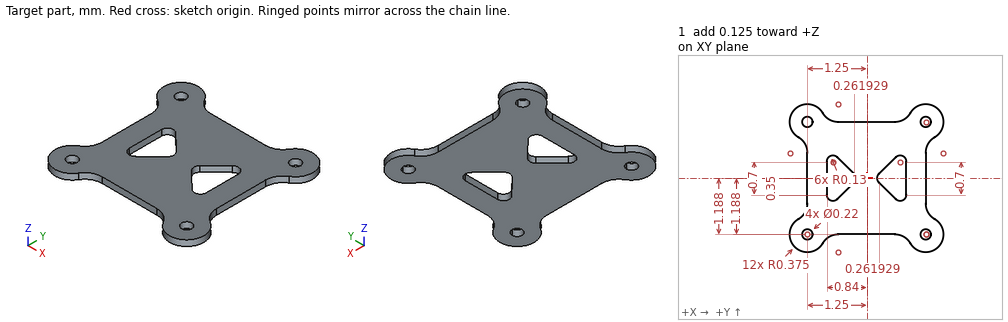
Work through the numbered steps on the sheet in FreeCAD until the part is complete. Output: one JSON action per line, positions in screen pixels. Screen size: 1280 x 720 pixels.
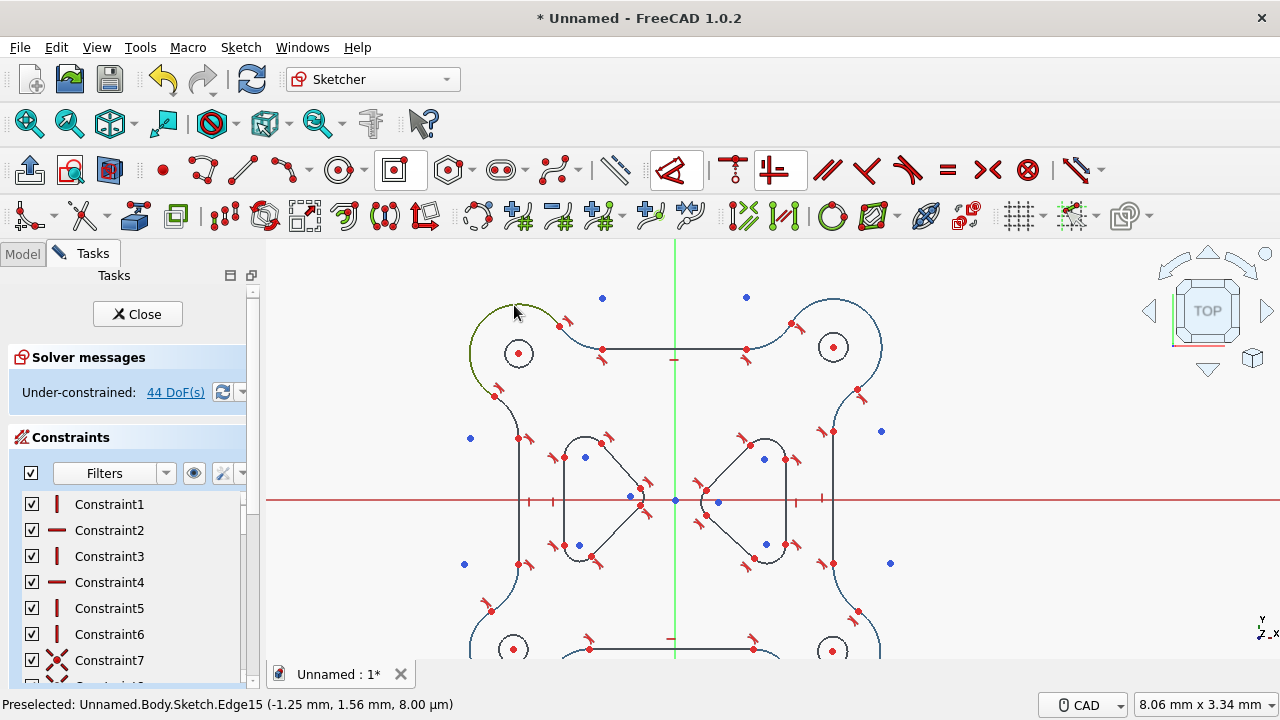
{"action": "left_click", "coordinate": [516, 423]}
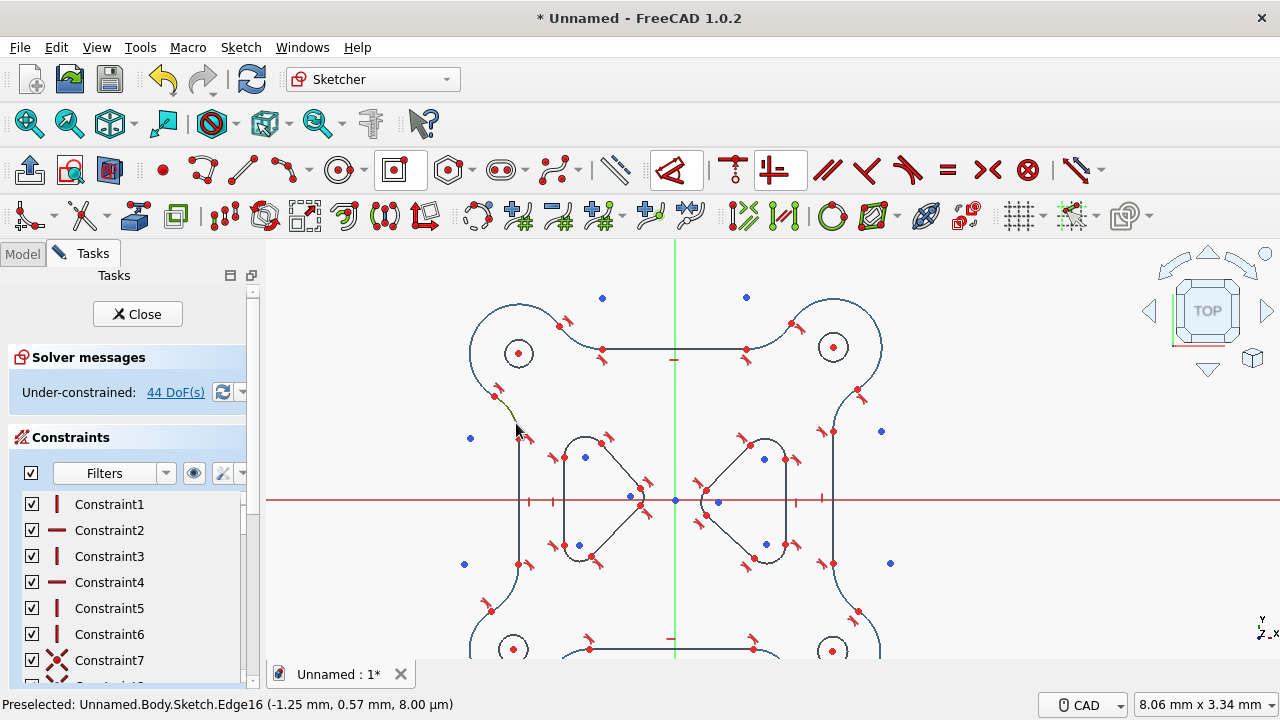
{"action": "left_click", "coordinate": [948, 170]}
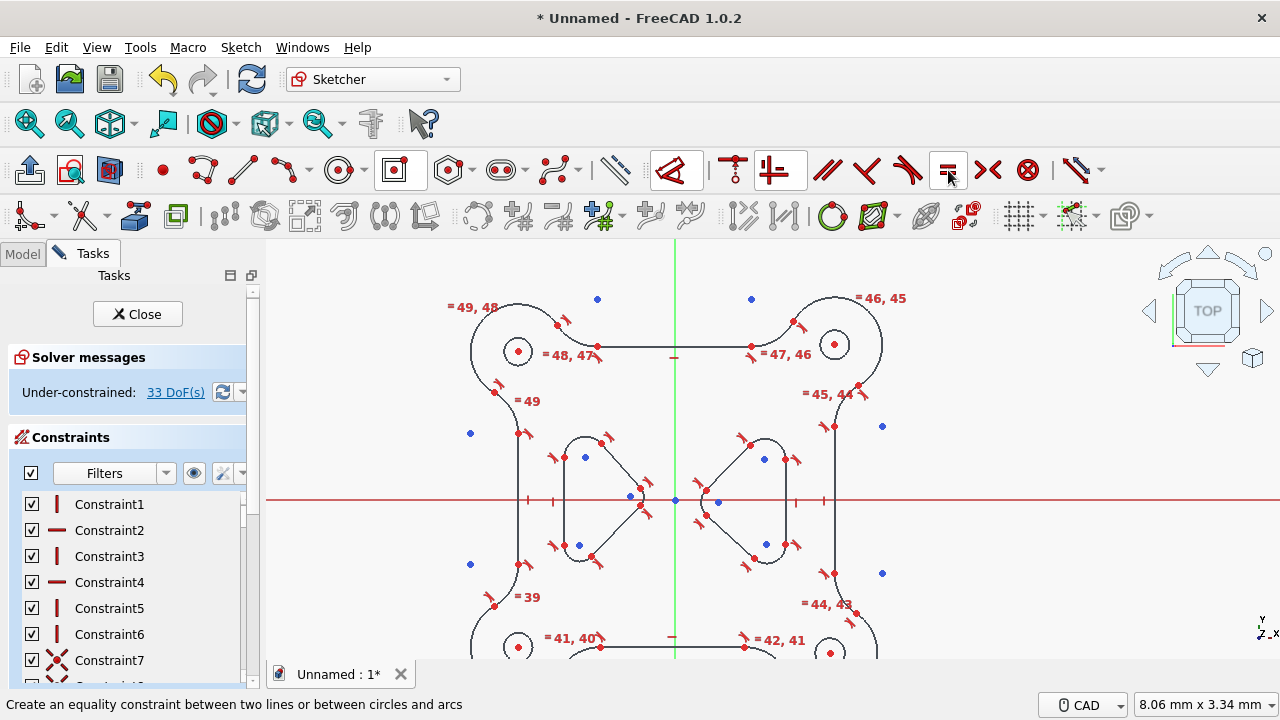
{"action": "left_click", "coordinate": [588, 437]}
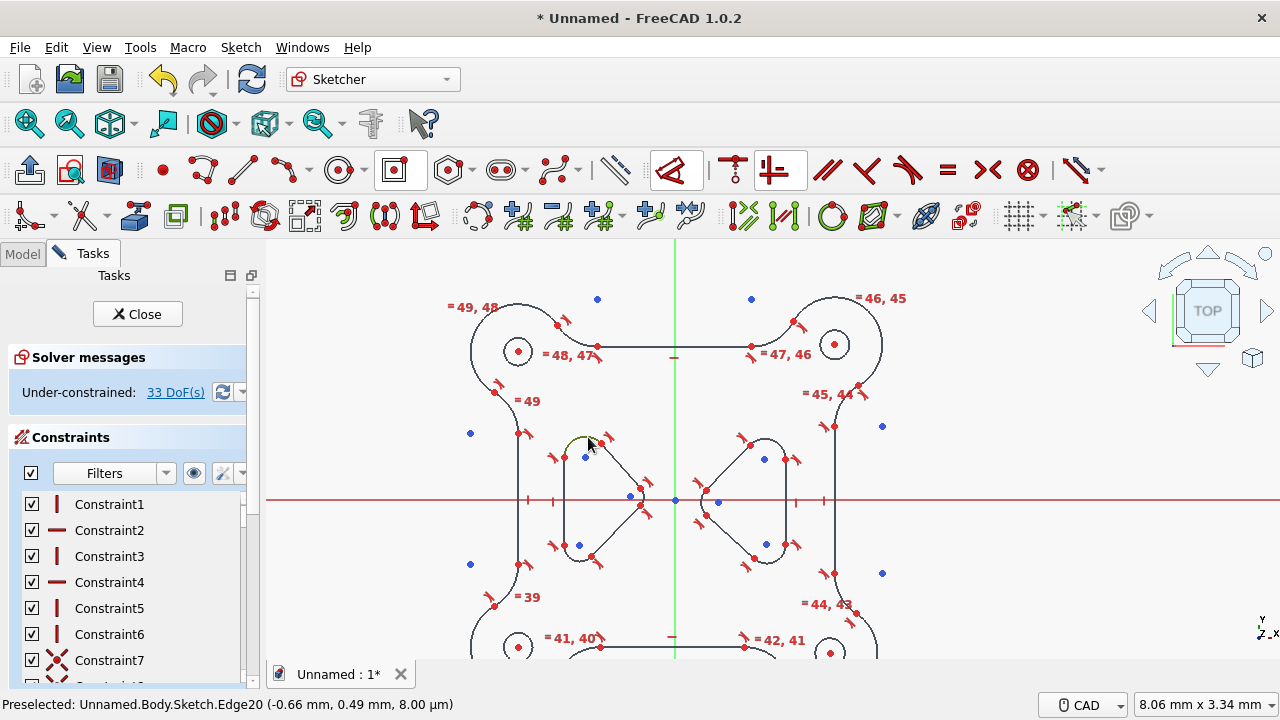
{"action": "scroll", "coordinate": [644, 497], "scroll_direction": "up", "scroll_amount": 2}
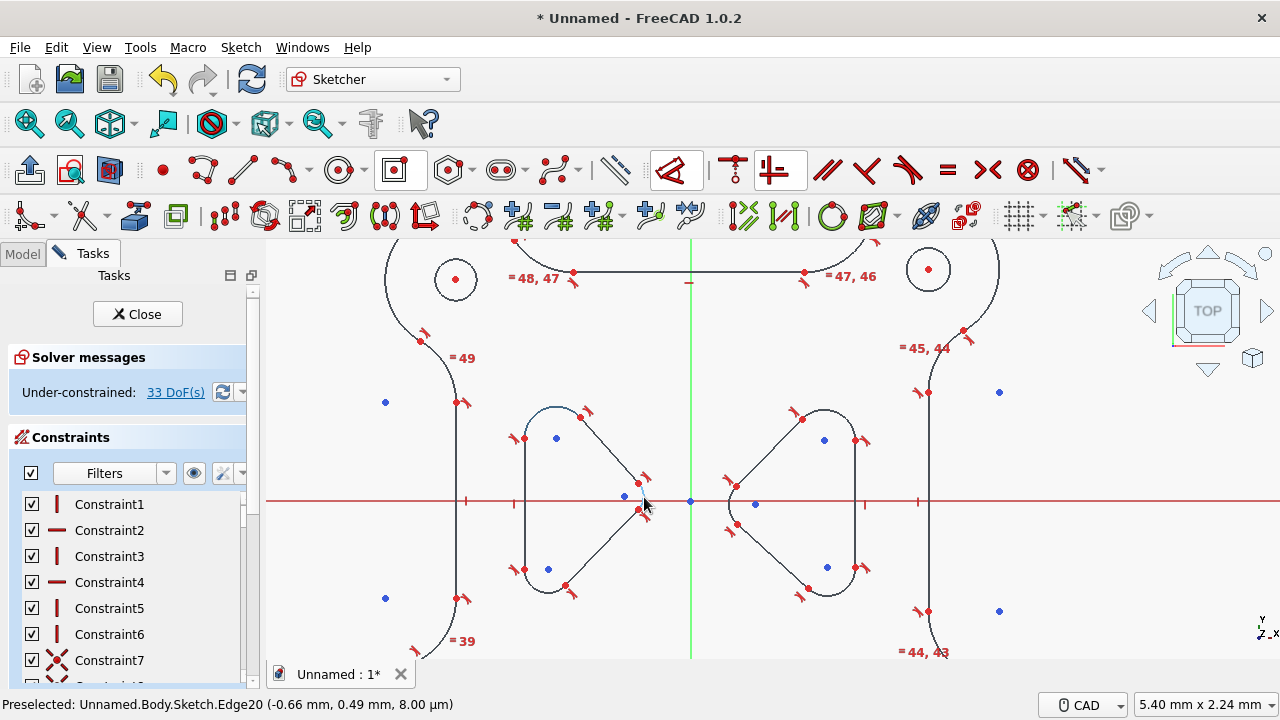
{"action": "left_click", "coordinate": [644, 497]}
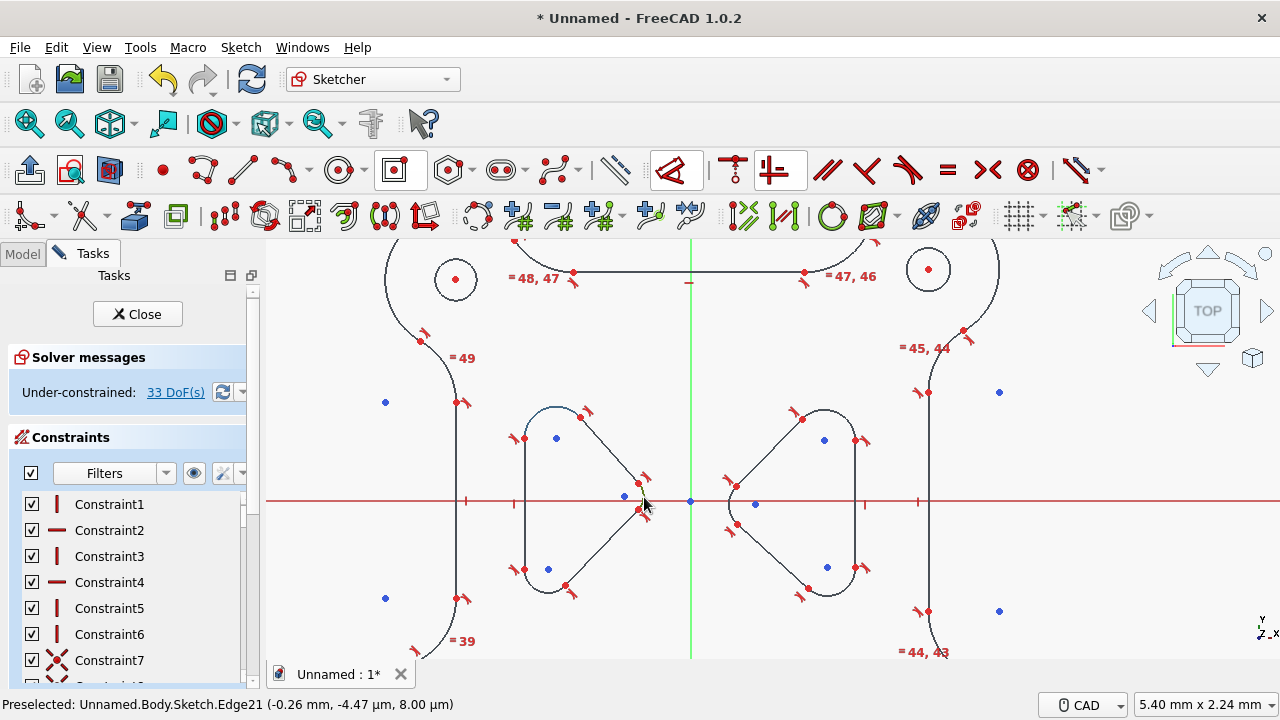
{"action": "left_click", "coordinate": [530, 585]}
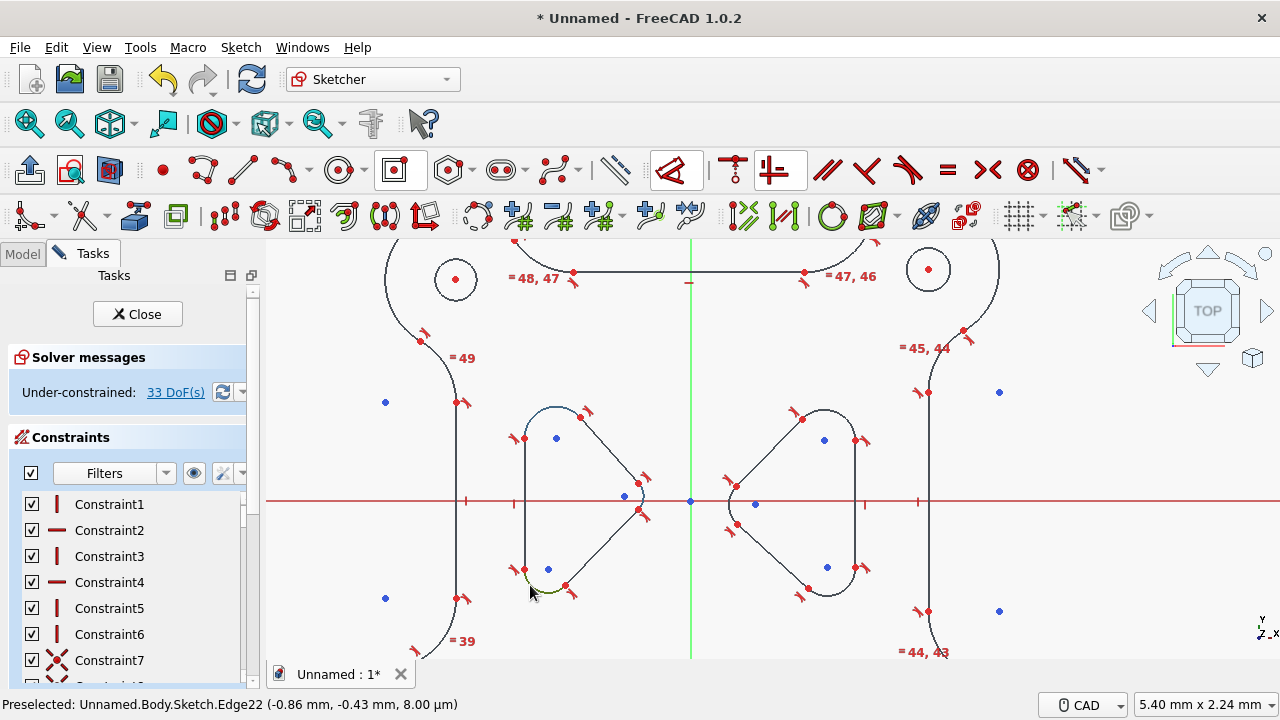
{"action": "left_click", "coordinate": [731, 514]}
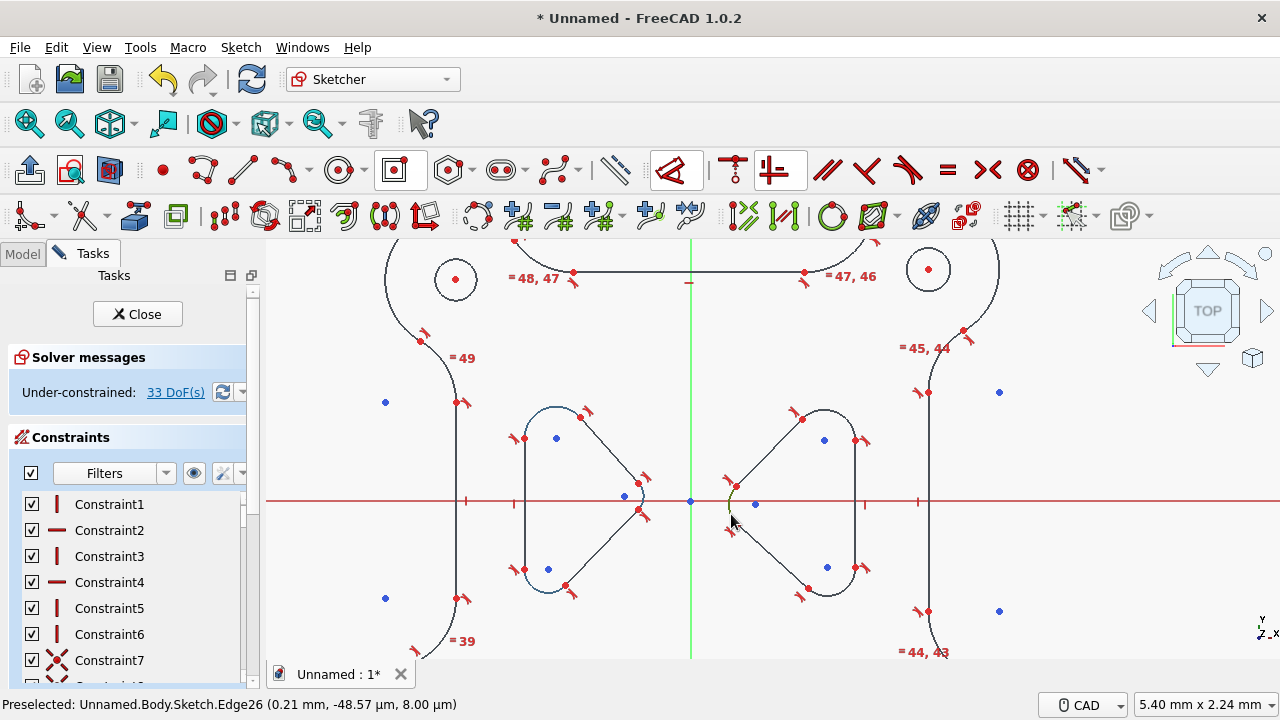
{"action": "left_click", "coordinate": [848, 421]}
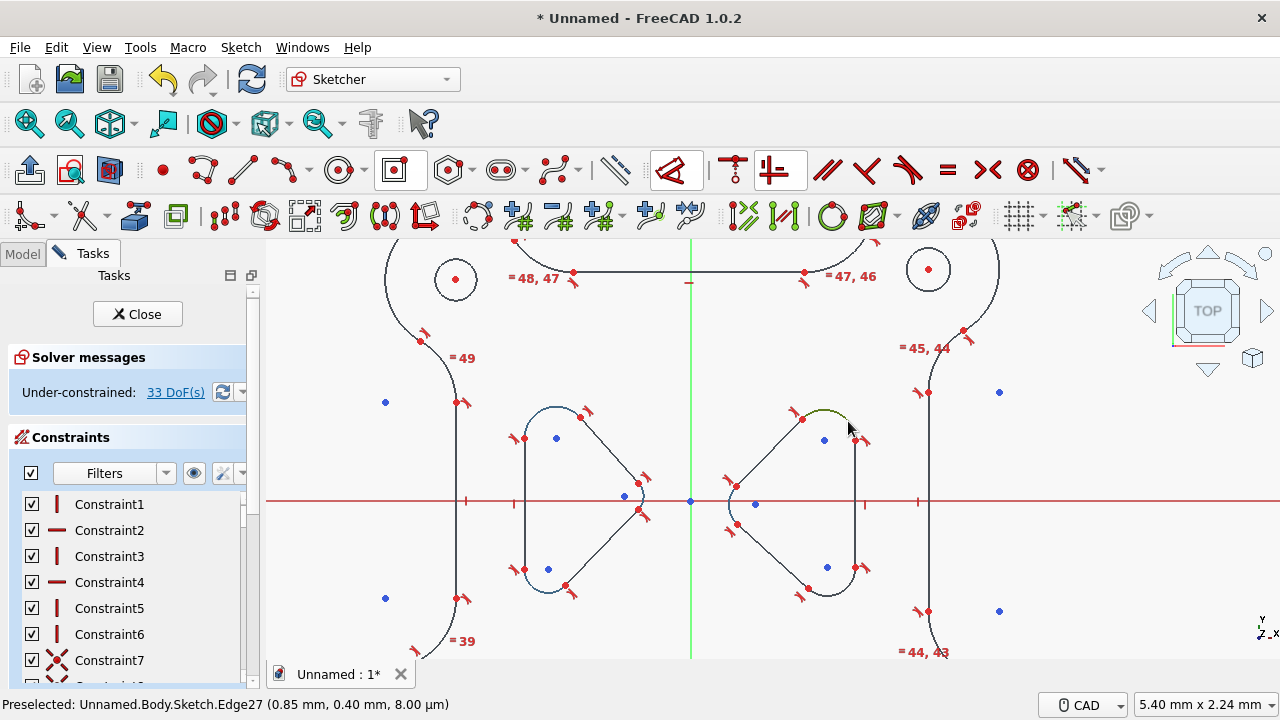
{"action": "left_click", "coordinate": [826, 596]}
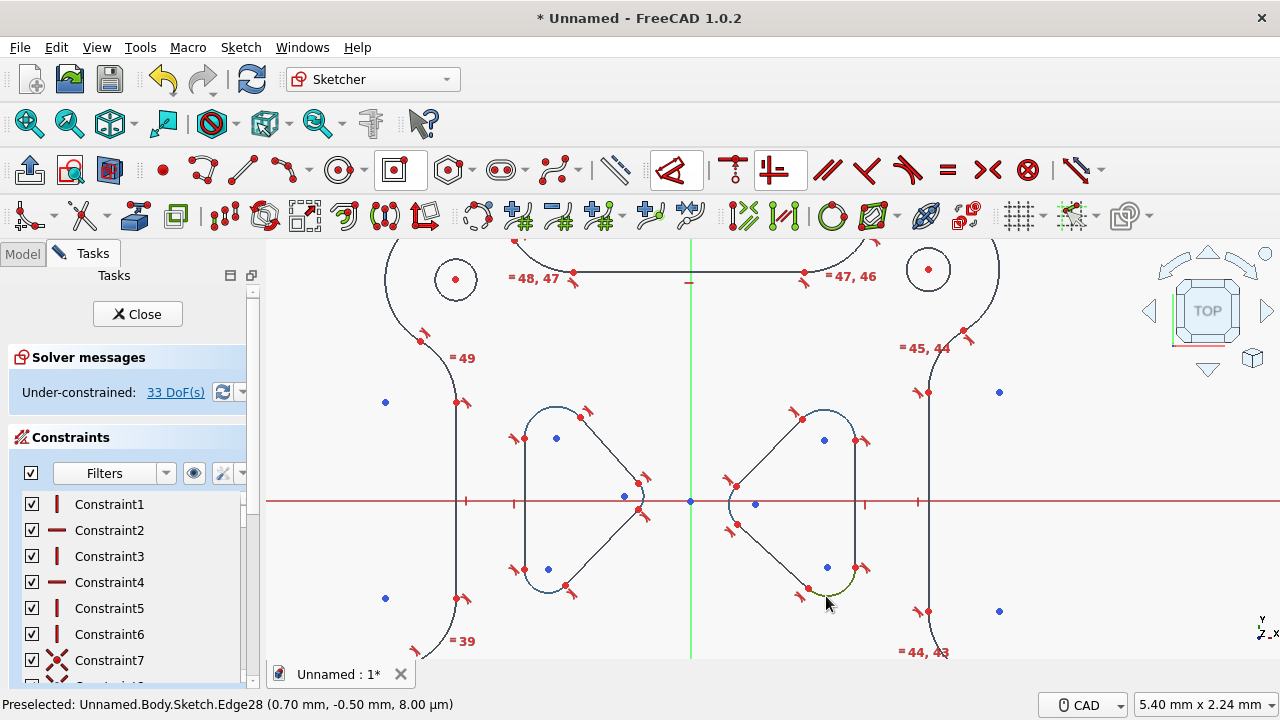
{"action": "left_click", "coordinate": [948, 170]}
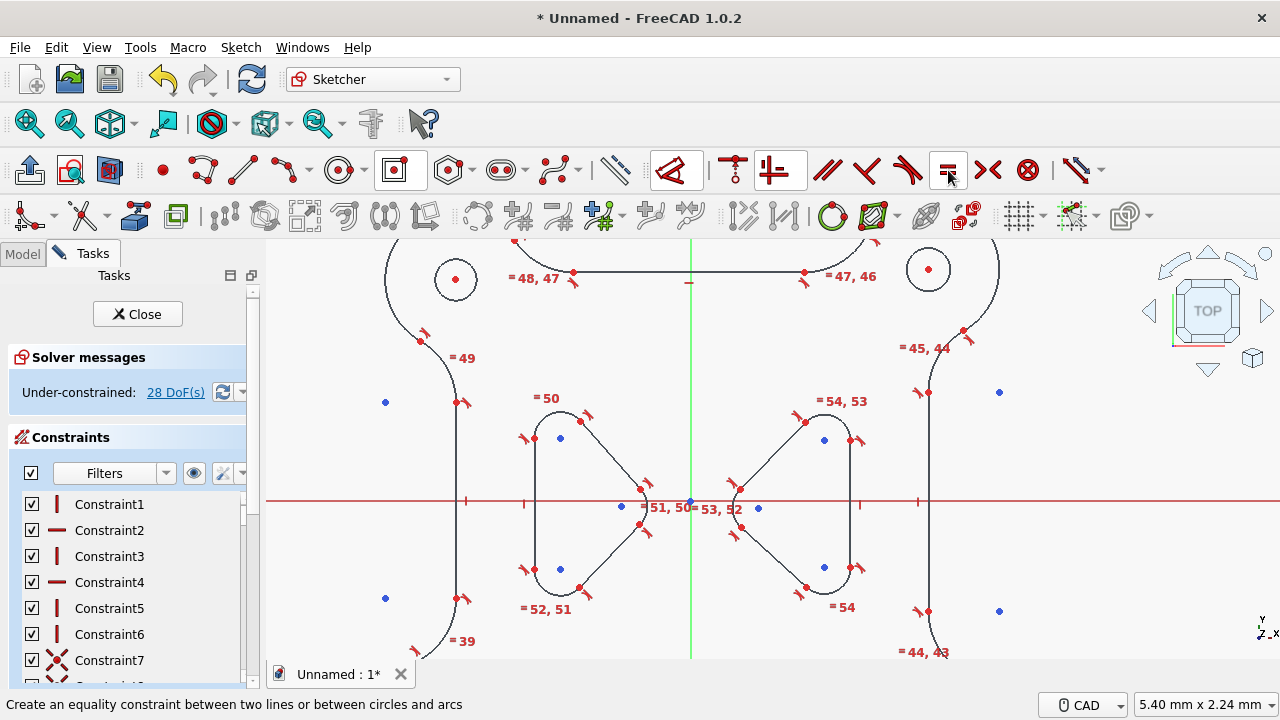
{"action": "scroll", "coordinate": [716, 406], "scroll_direction": "down", "scroll_amount": 4}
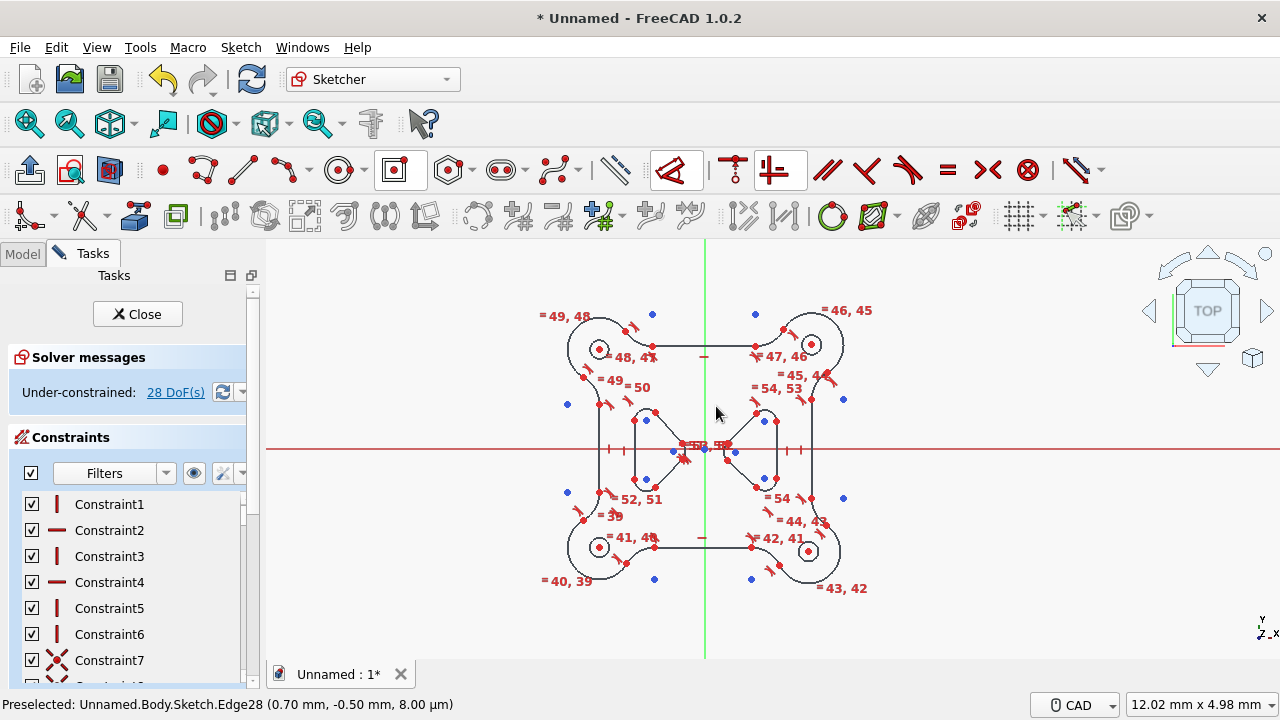
{"action": "scroll", "coordinate": [606, 541], "scroll_direction": "up", "scroll_amount": 2}